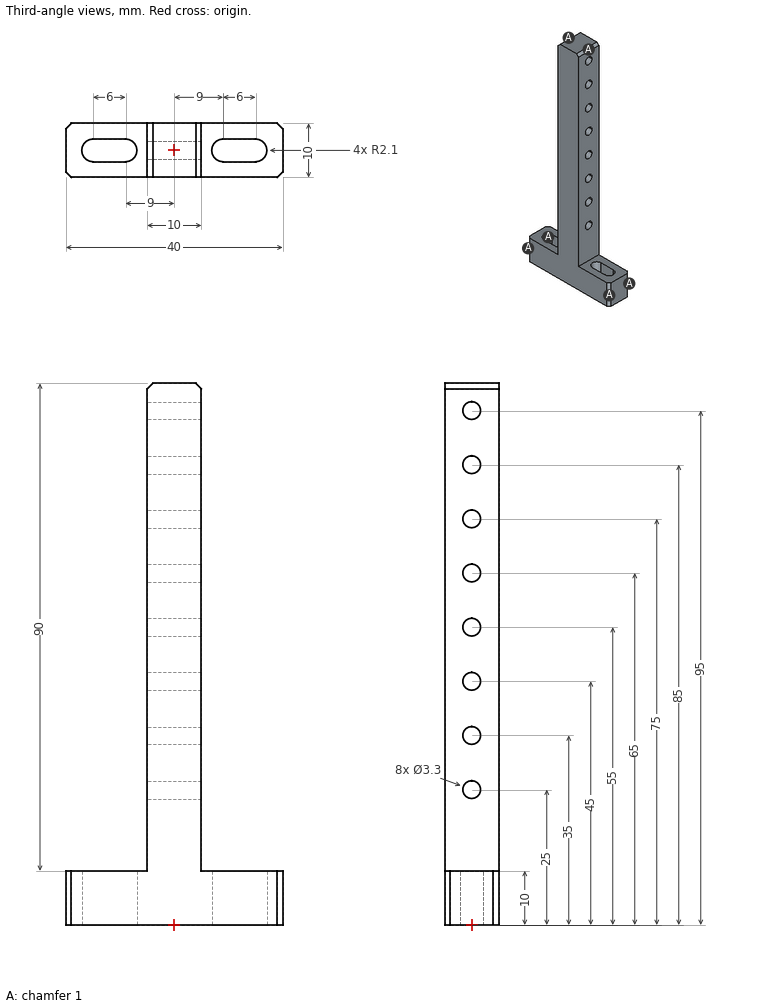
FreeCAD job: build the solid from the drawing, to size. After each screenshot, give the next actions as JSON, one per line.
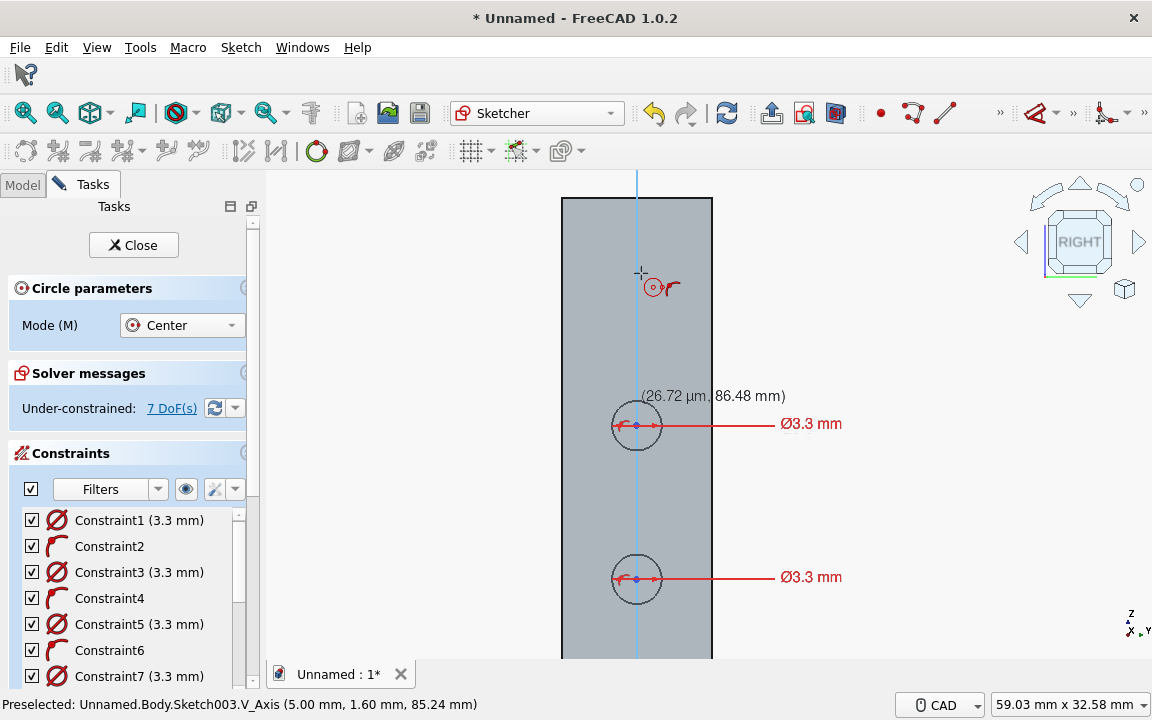
{"action": "scroll", "coordinate": [641, 273], "scroll_direction": "down", "scroll_amount": 8}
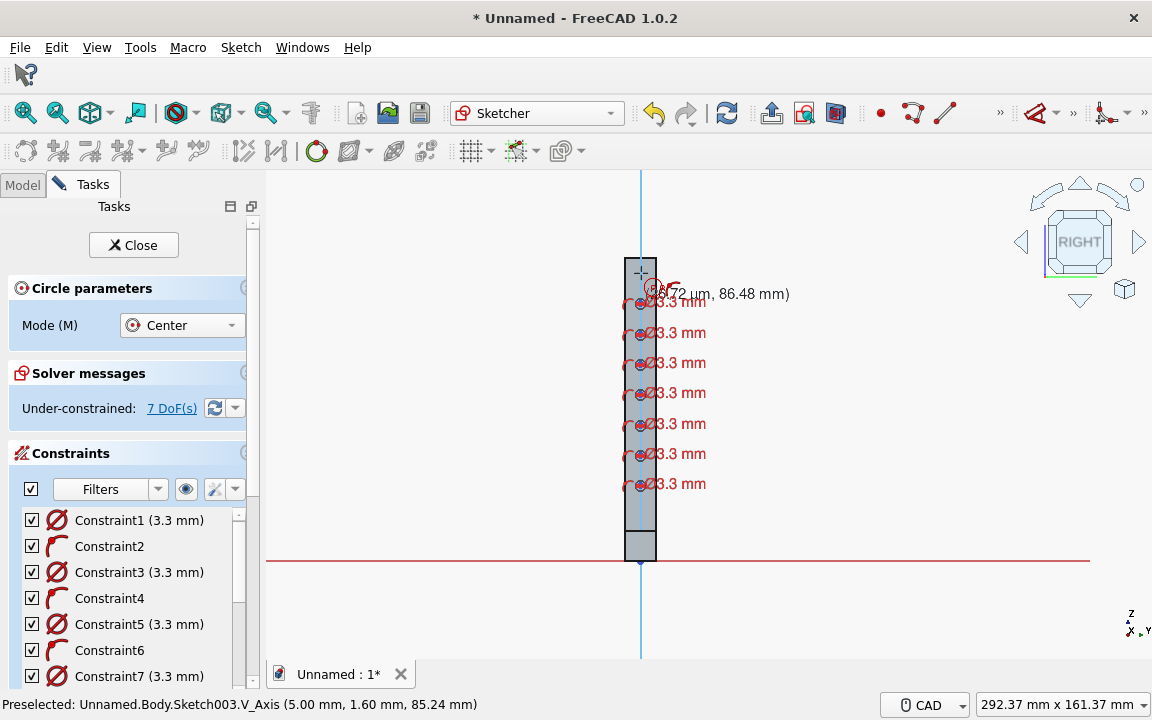
{"action": "left_click", "coordinate": [641, 273]}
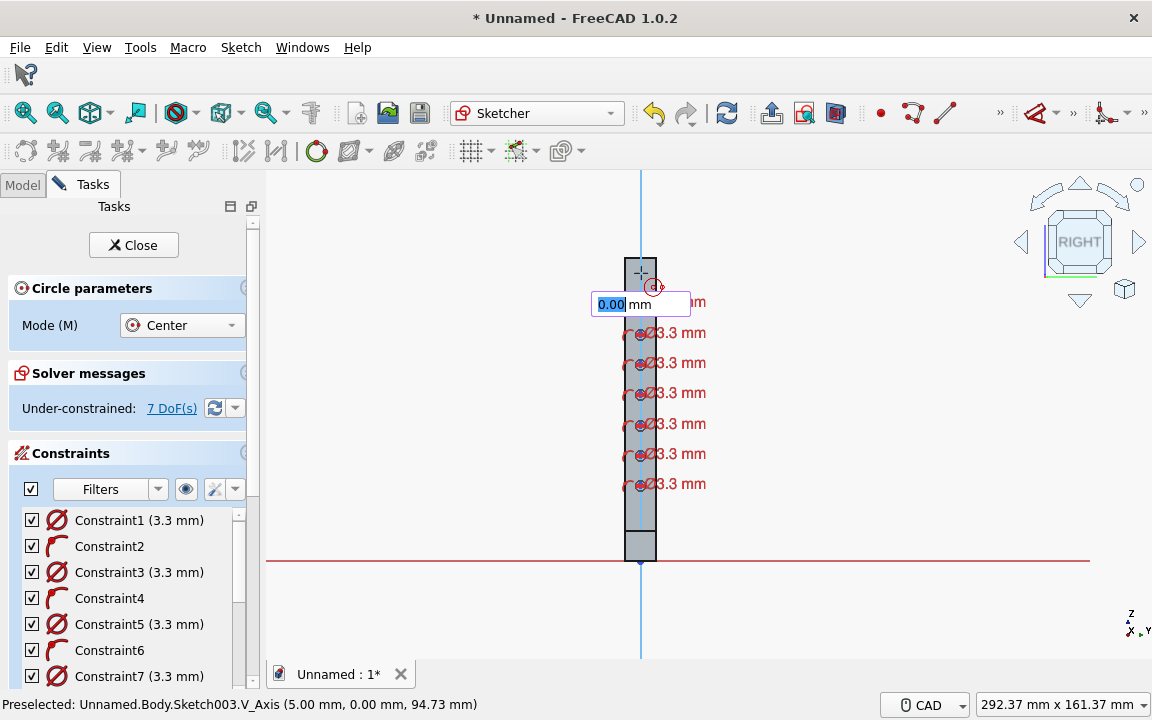
{"action": "scroll", "coordinate": [645, 271], "scroll_direction": "up", "scroll_amount": 7}
{"action": "mouse_move", "coordinate": [645, 272]}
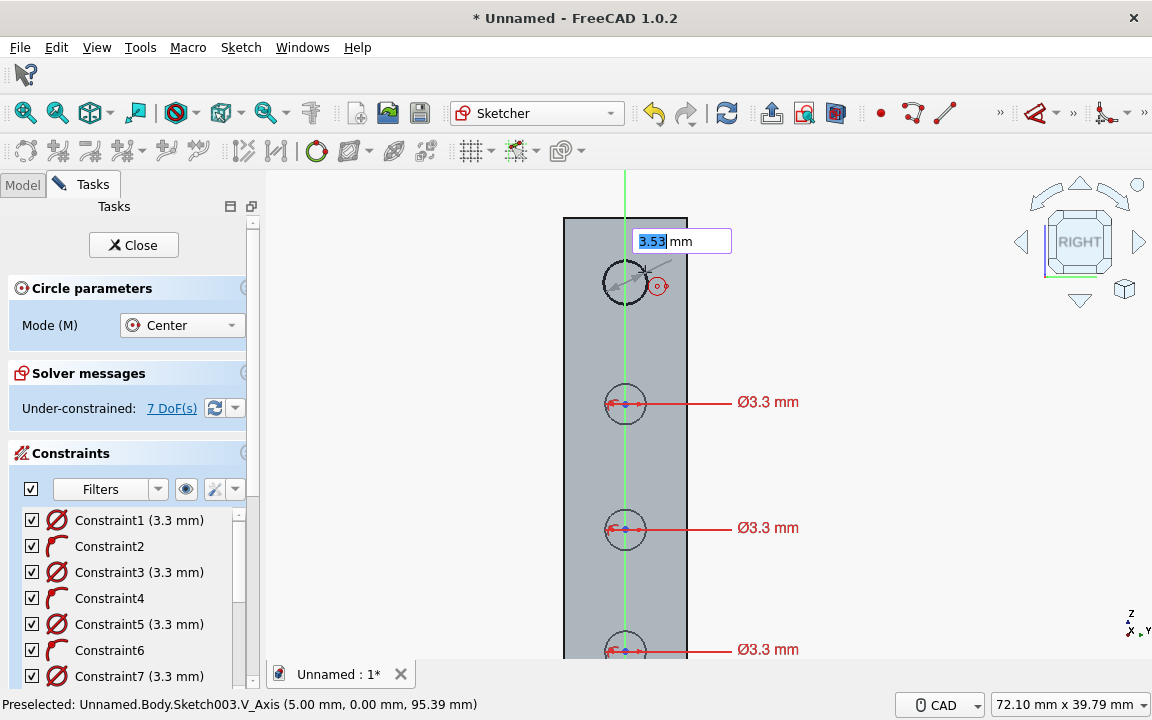
{"action": "type", "text": "3.3"}
{"action": "key", "text": "Return"}
{"action": "key", "text": "Escape"}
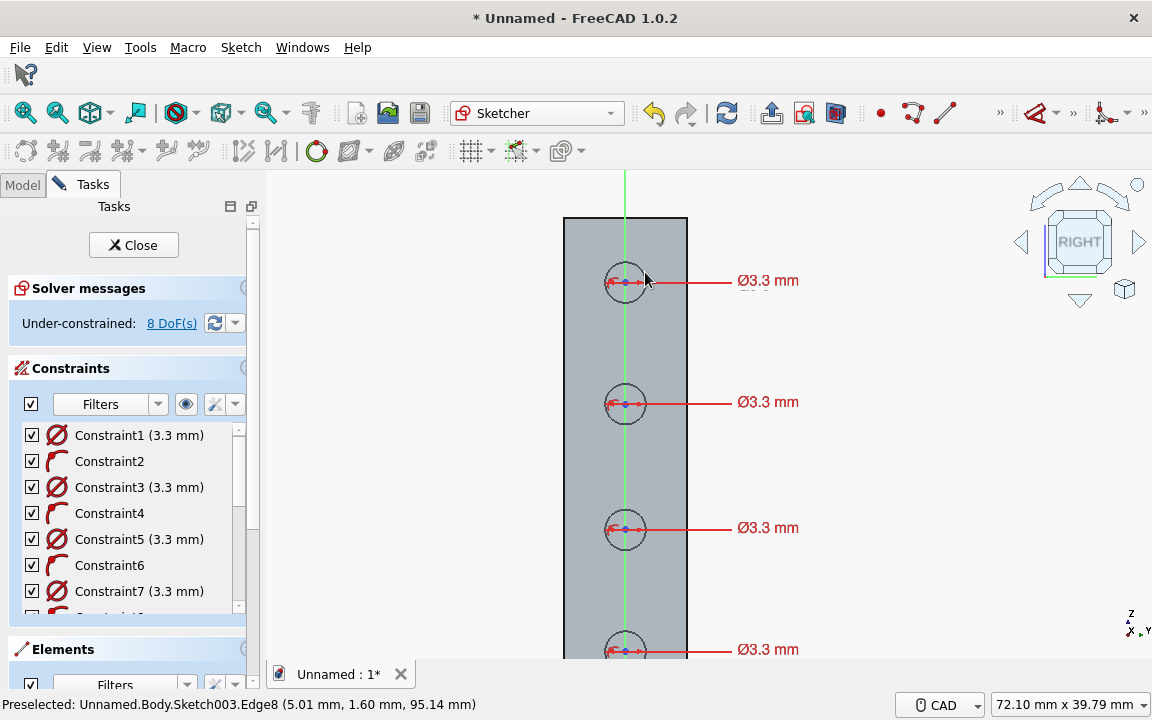
{"action": "left_click", "coordinate": [1036, 114]}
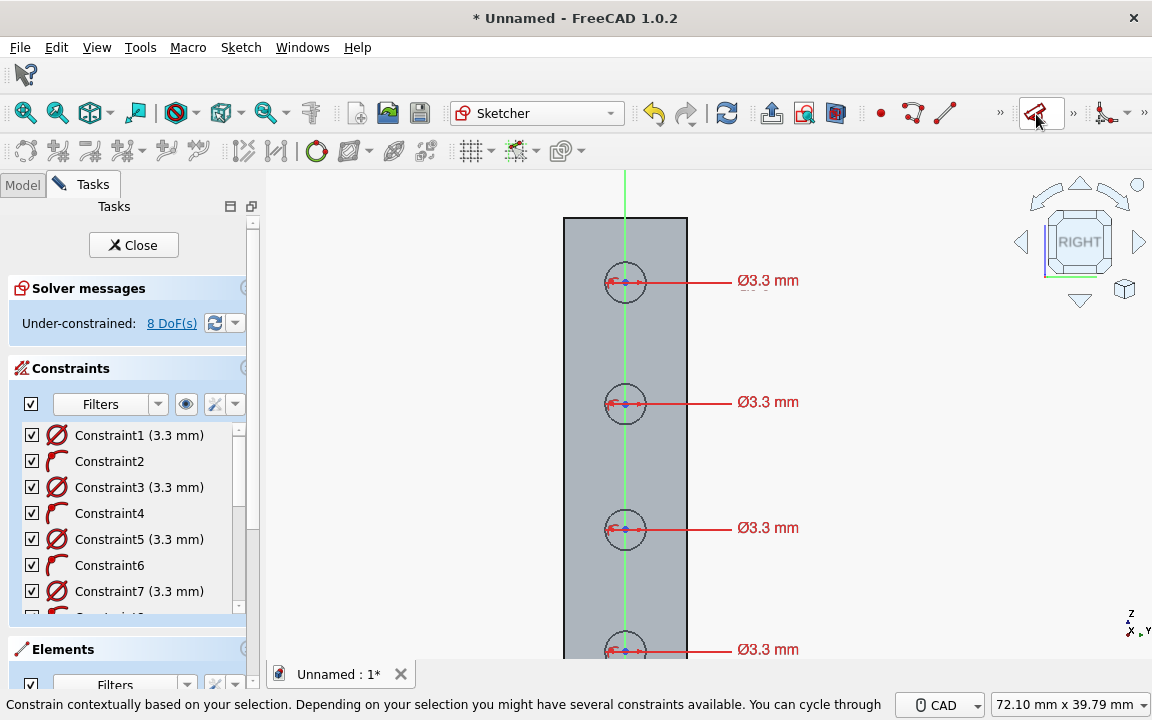
{"action": "scroll", "coordinate": [645, 271], "scroll_direction": "down", "scroll_amount": 7}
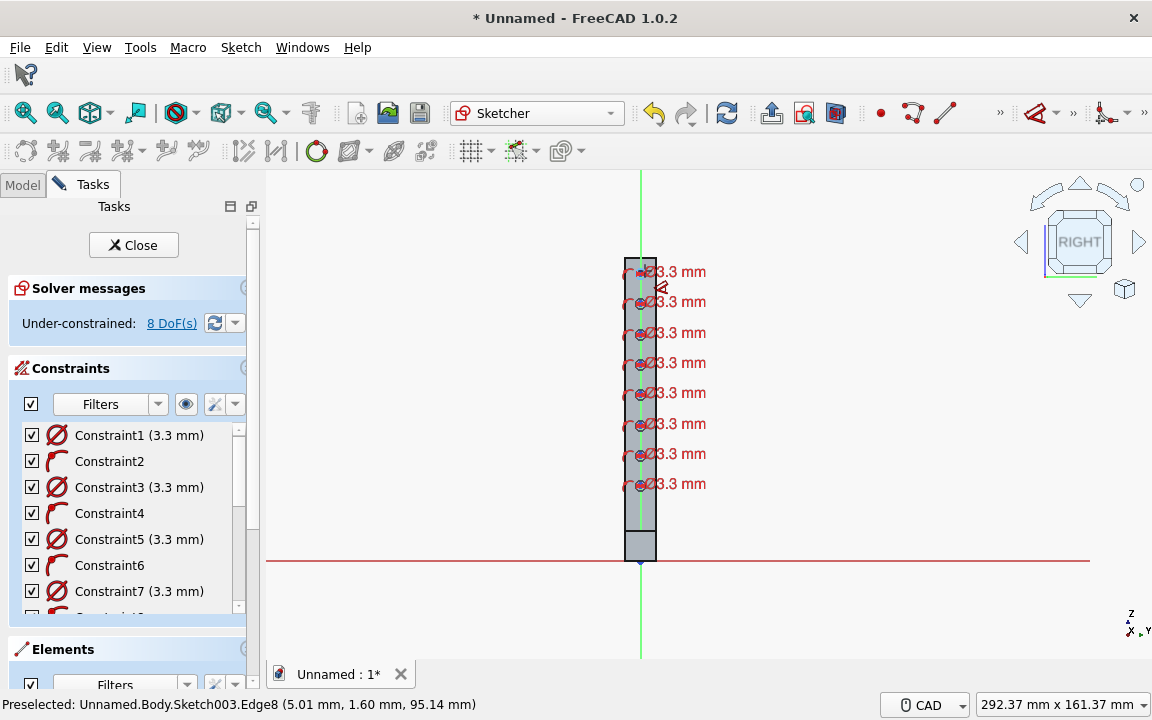
{"action": "left_click", "coordinate": [641, 486]}
{"action": "left_click", "coordinate": [675, 524]}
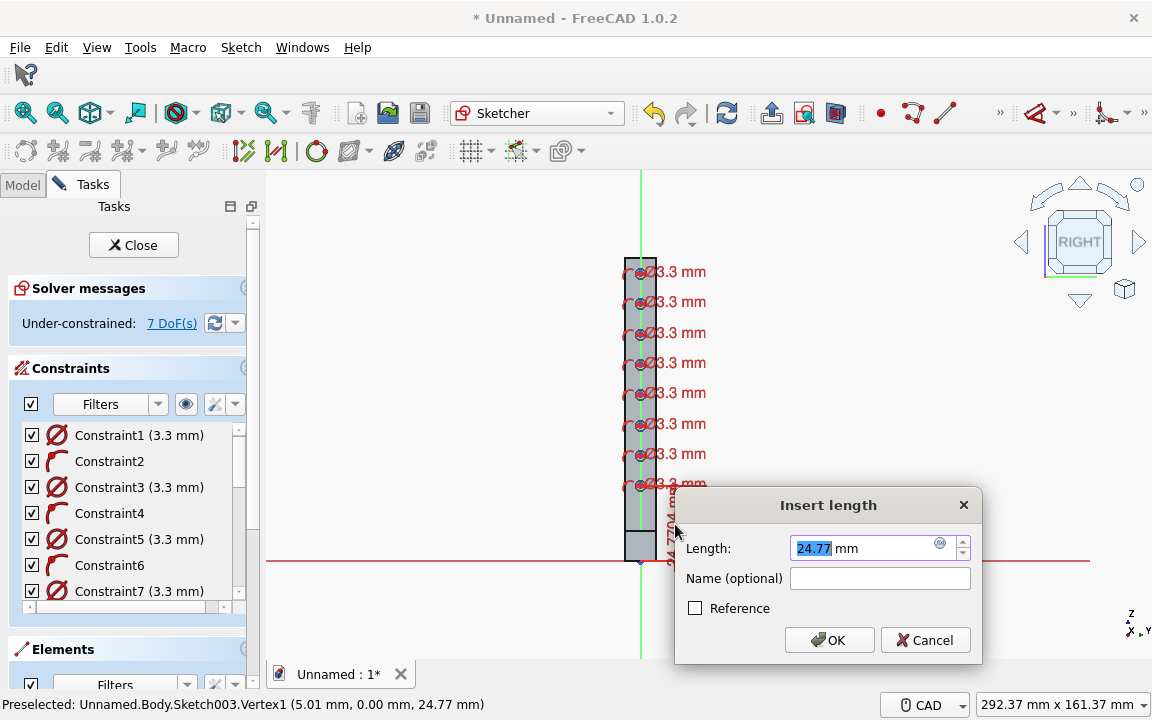
{"action": "type", "text": "25"}
{"action": "key", "text": "Return"}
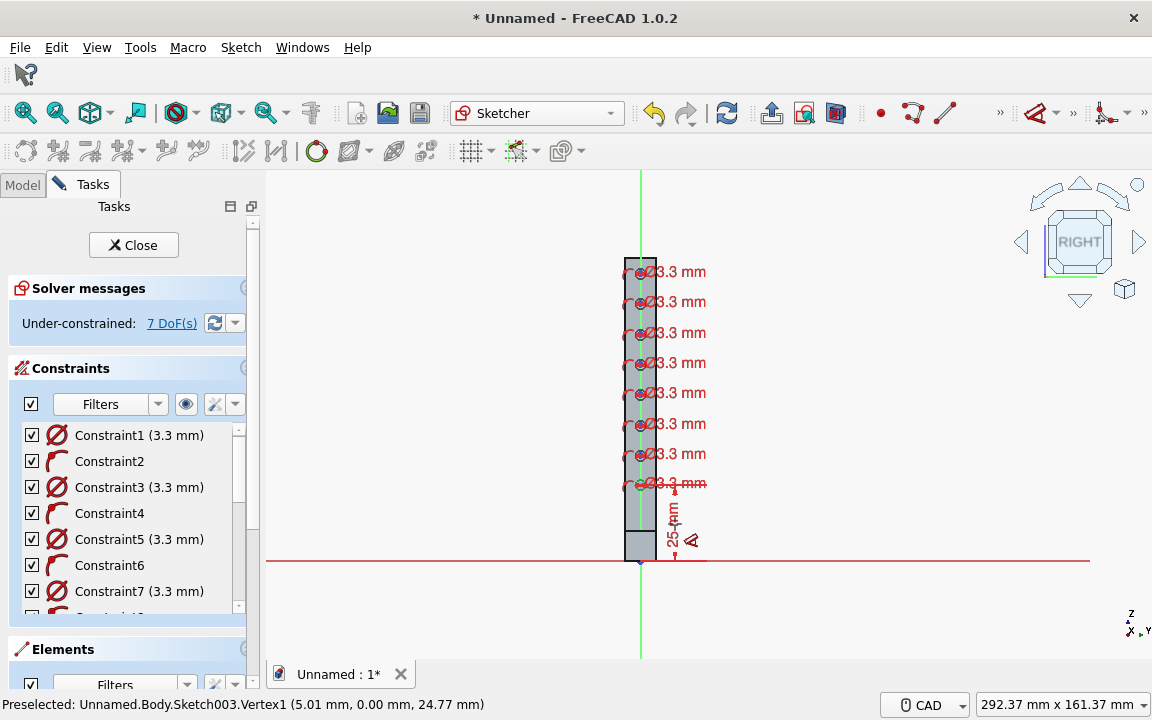
{"action": "left_click", "coordinate": [641, 456]}
{"action": "left_click", "coordinate": [675, 484]}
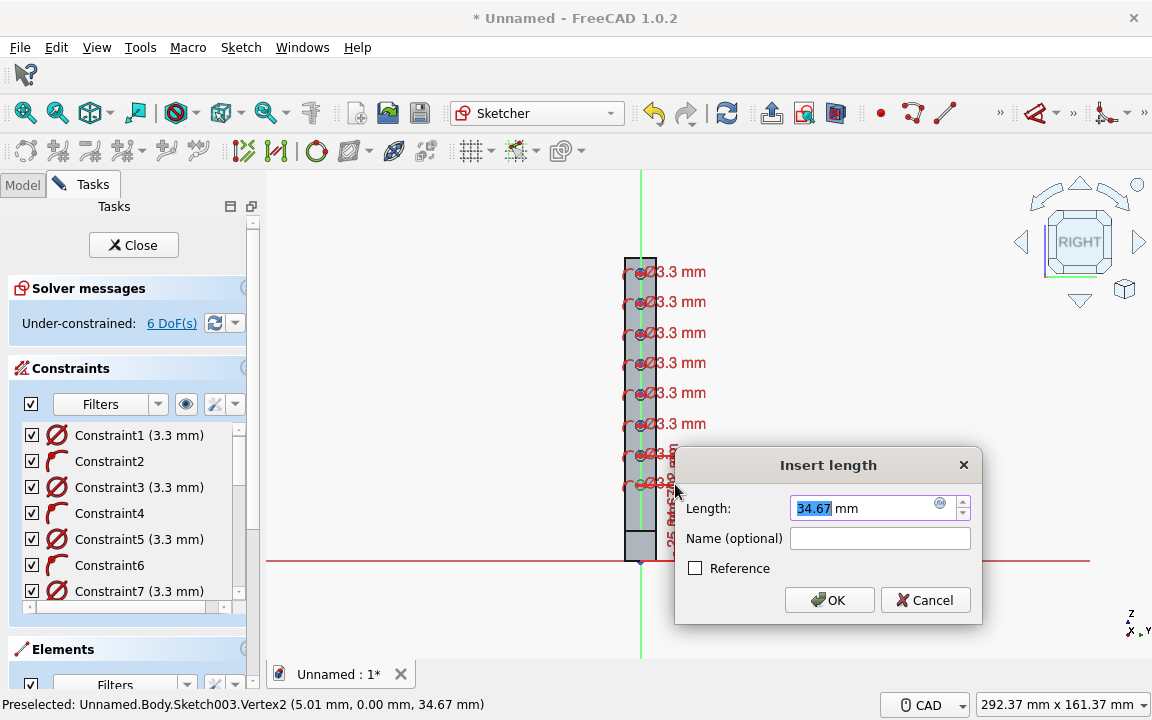
{"action": "type", "text": "35"}
{"action": "key", "text": "Return"}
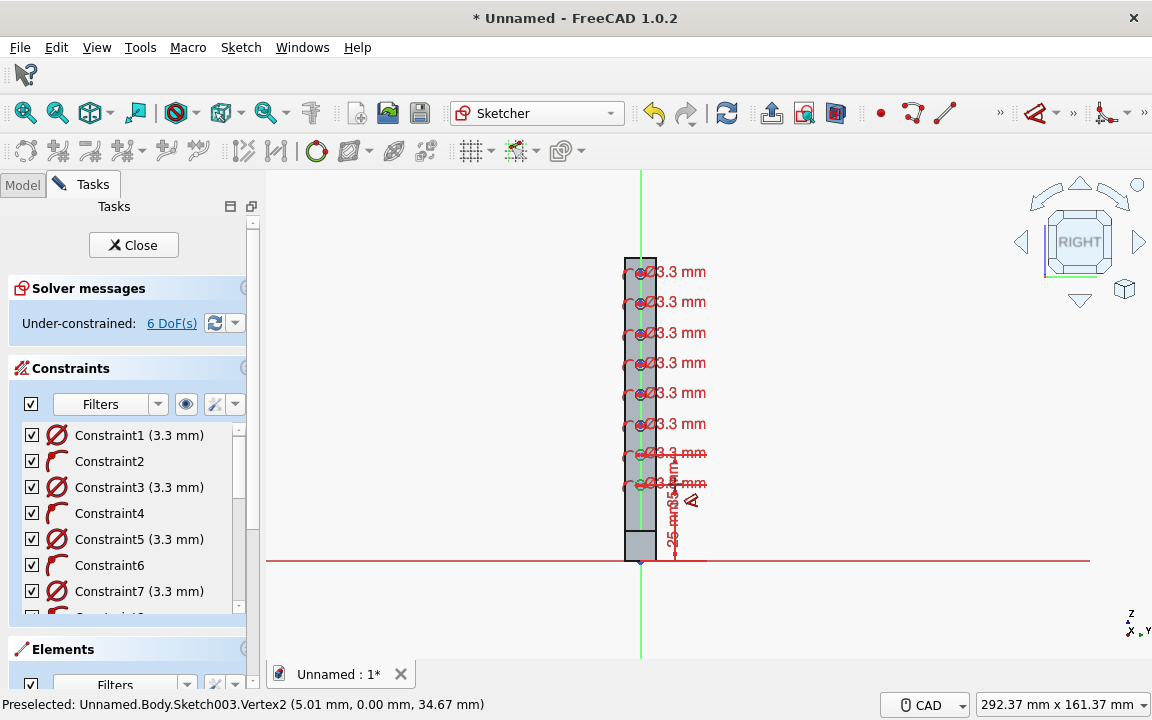
{"action": "left_click", "coordinate": [641, 426]}
{"action": "left_click", "coordinate": [675, 462]}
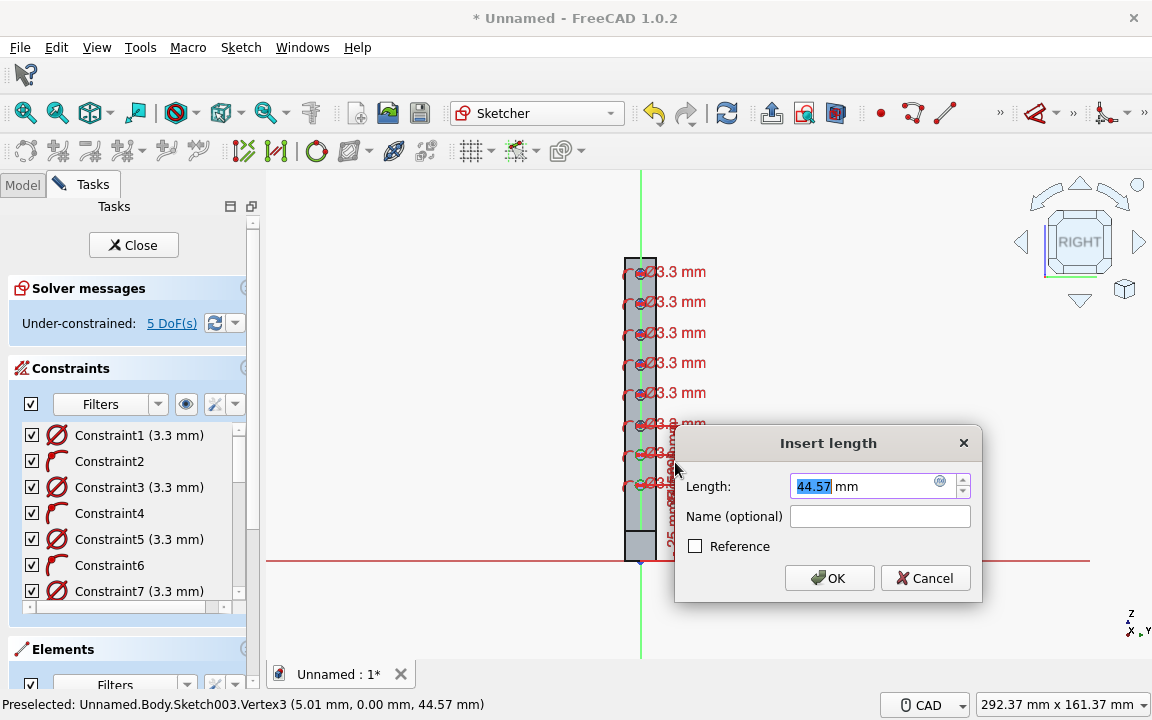
{"action": "type", "text": "45"}
{"action": "key", "text": "Return"}